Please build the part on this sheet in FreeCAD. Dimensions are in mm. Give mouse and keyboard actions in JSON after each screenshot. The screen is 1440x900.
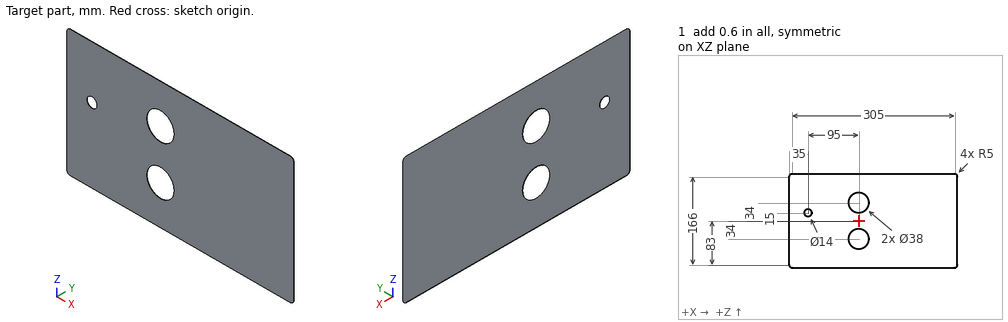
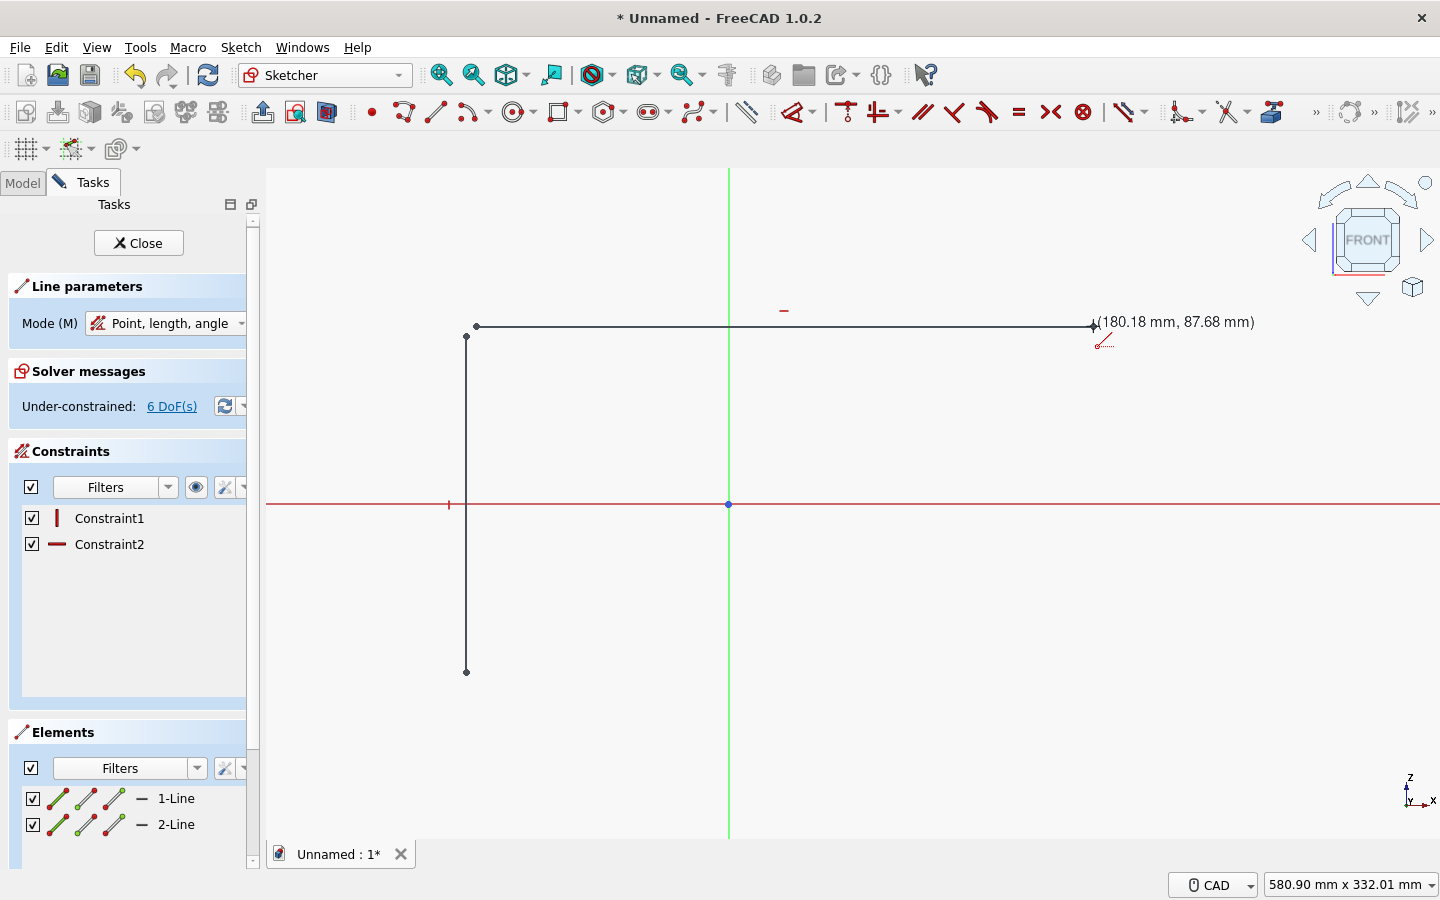
{"action": "left_click", "coordinate": [1103, 336]}
{"action": "left_click", "coordinate": [1103, 672]}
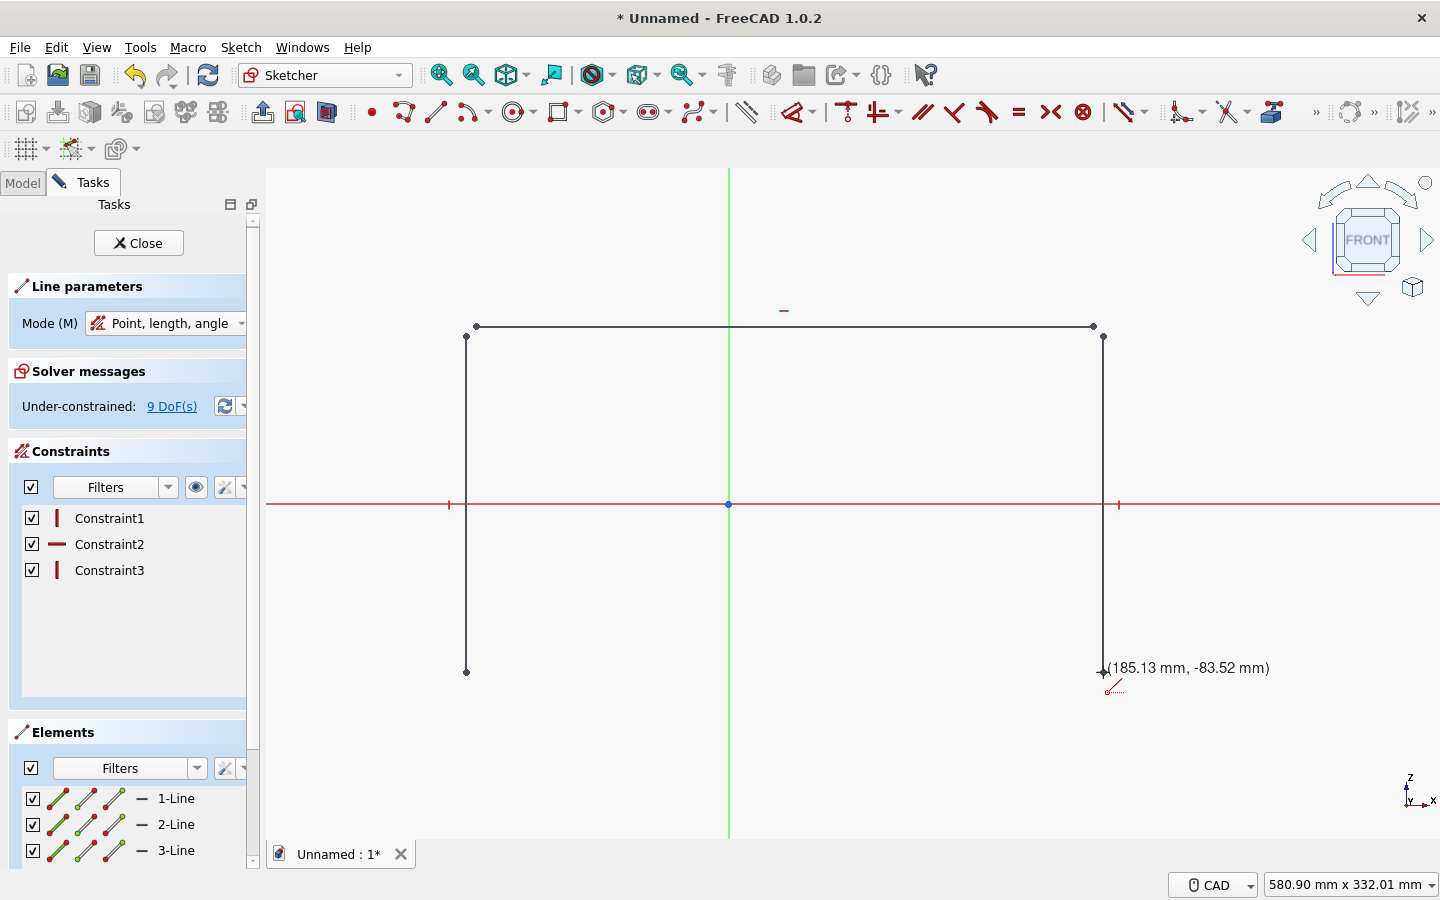
{"action": "left_click", "coordinate": [1093, 682]}
{"action": "left_click", "coordinate": [476, 682]}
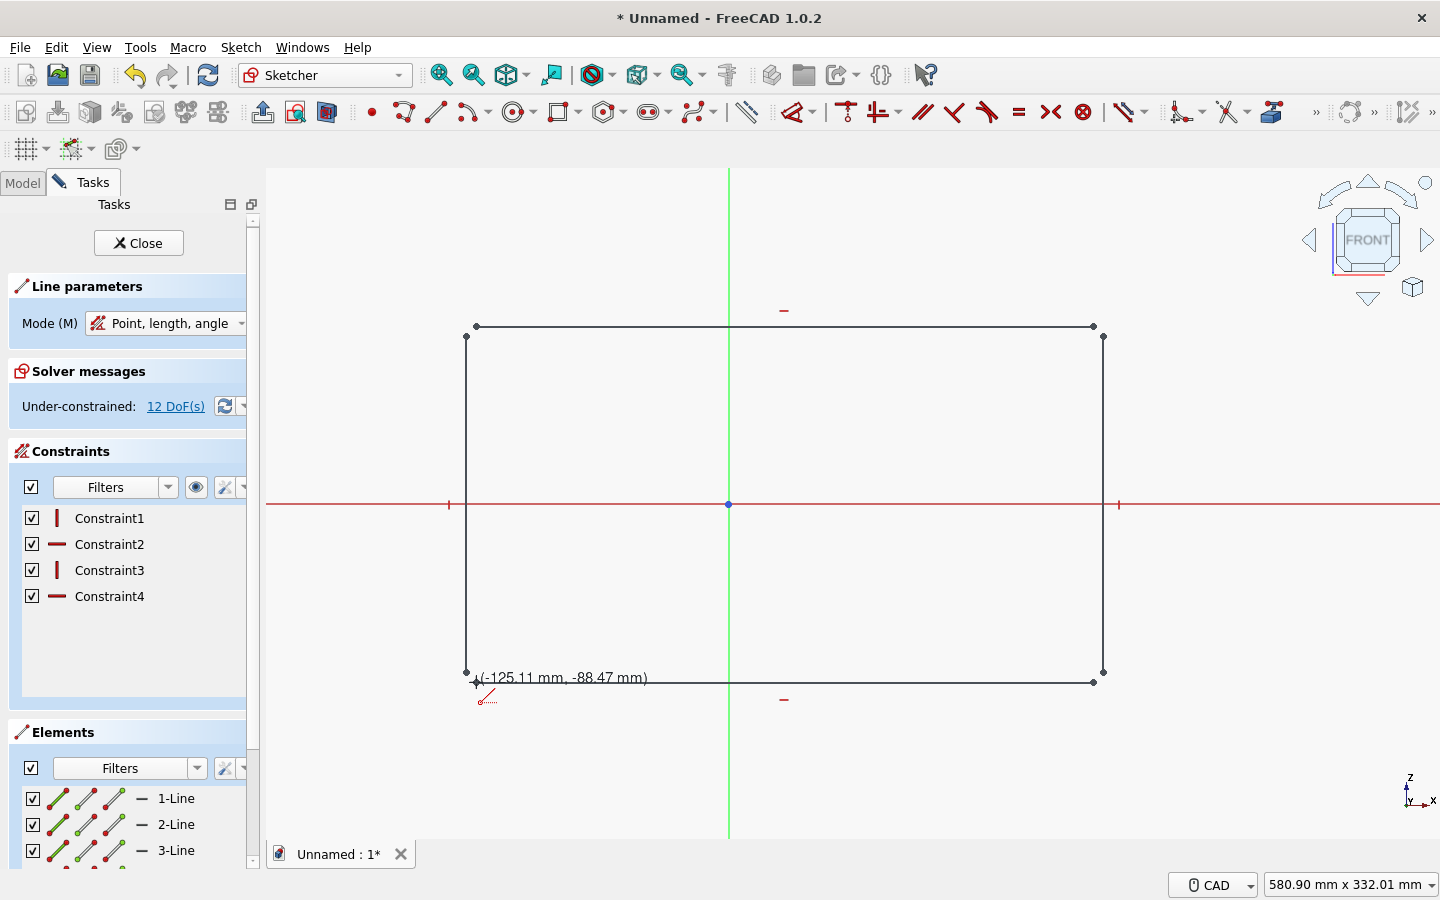
{"action": "left_click", "coordinate": [490, 112]}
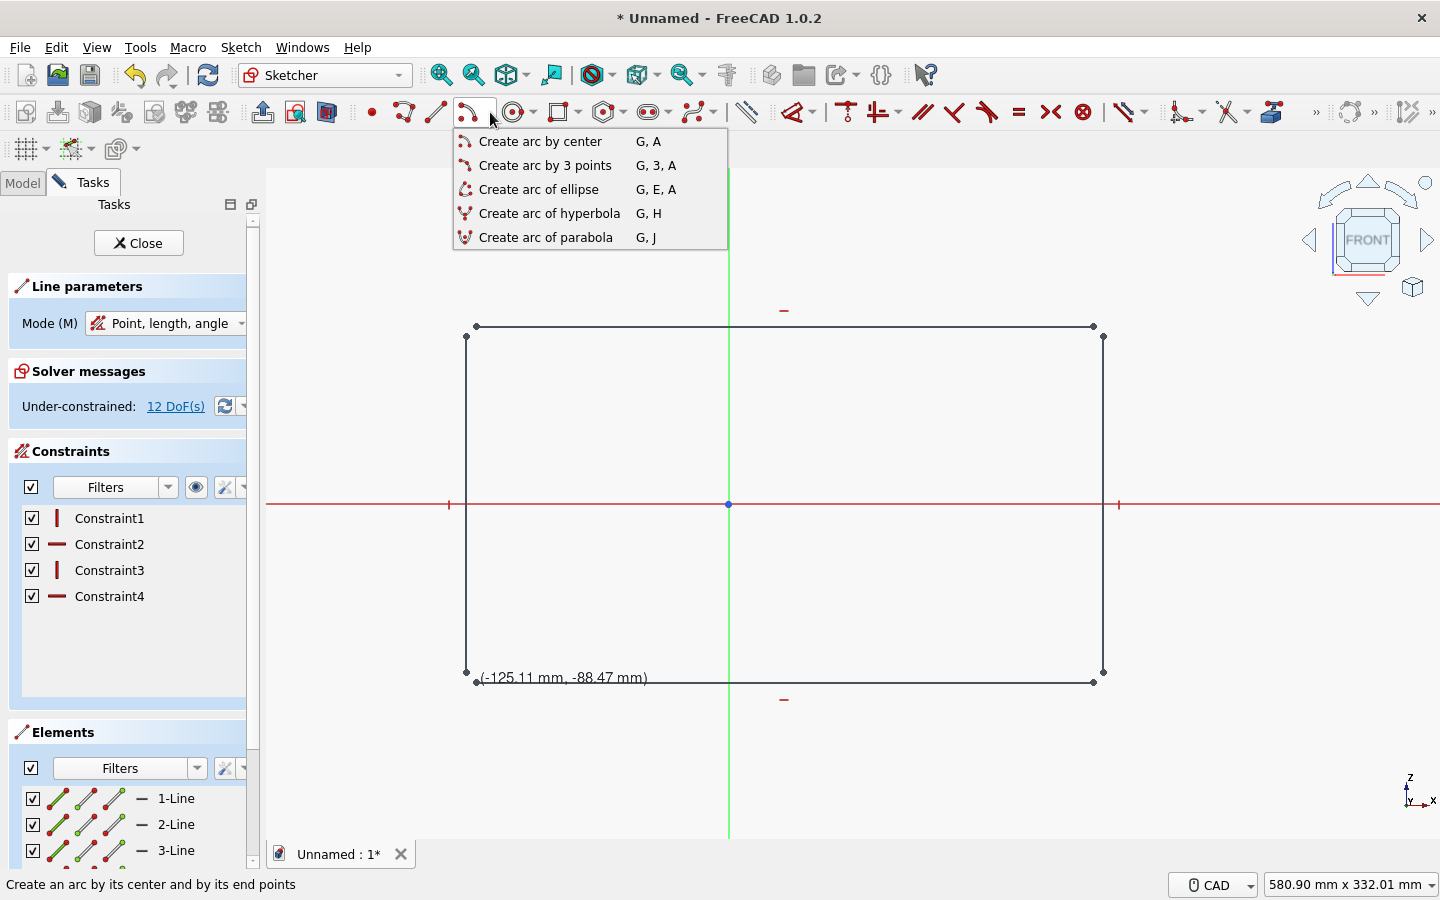
{"action": "left_click", "coordinate": [590, 165]}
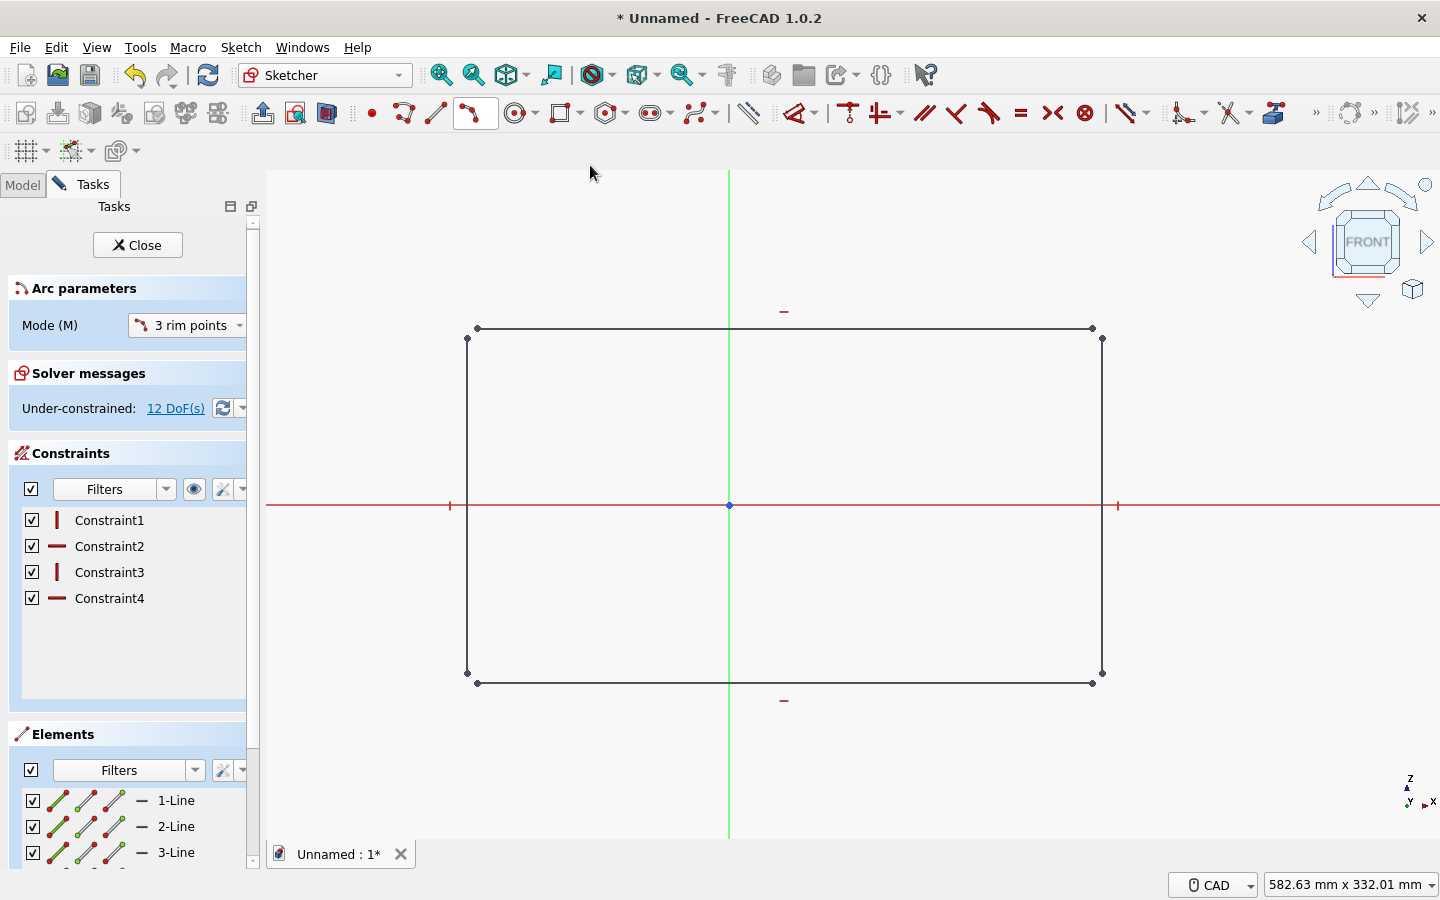
{"action": "left_click", "coordinate": [467, 338]}
{"action": "left_click", "coordinate": [477, 329]}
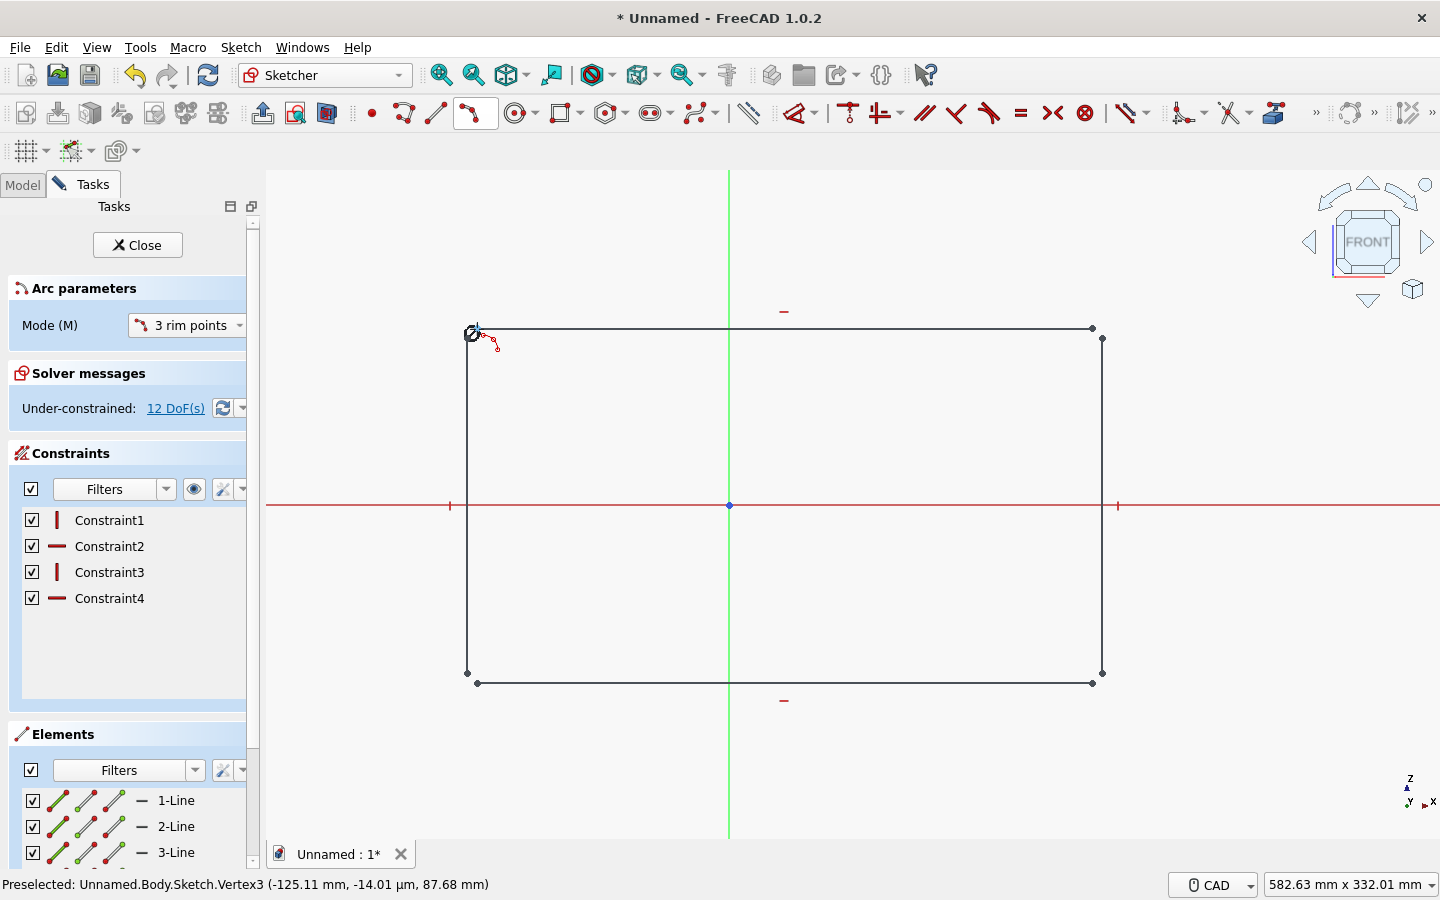
{"action": "scroll", "coordinate": [470, 331], "scroll_direction": "up", "scroll_amount": 9}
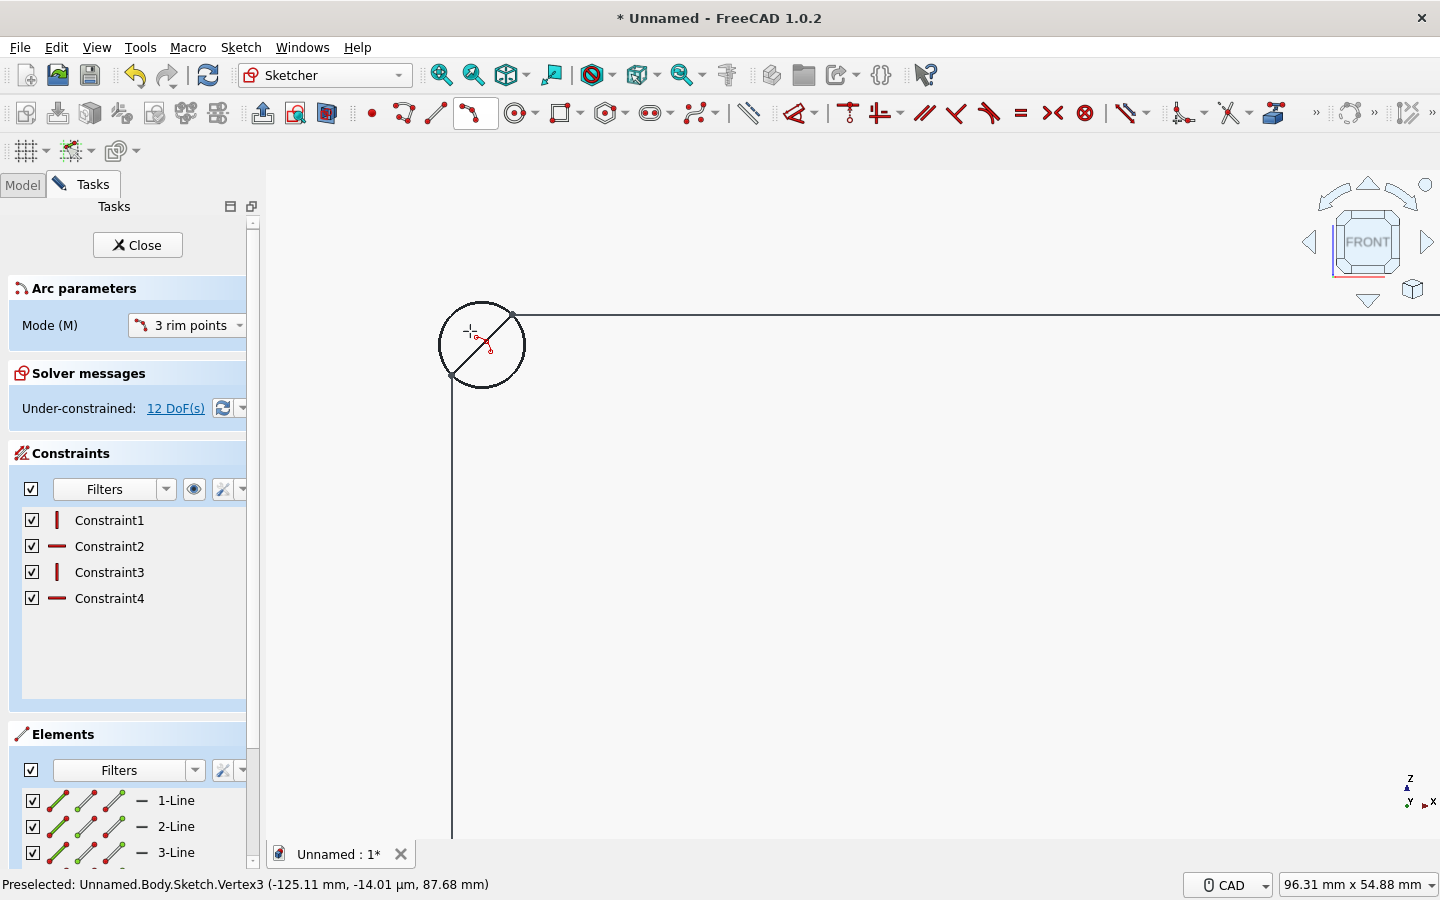
{"action": "left_click", "coordinate": [471, 329]}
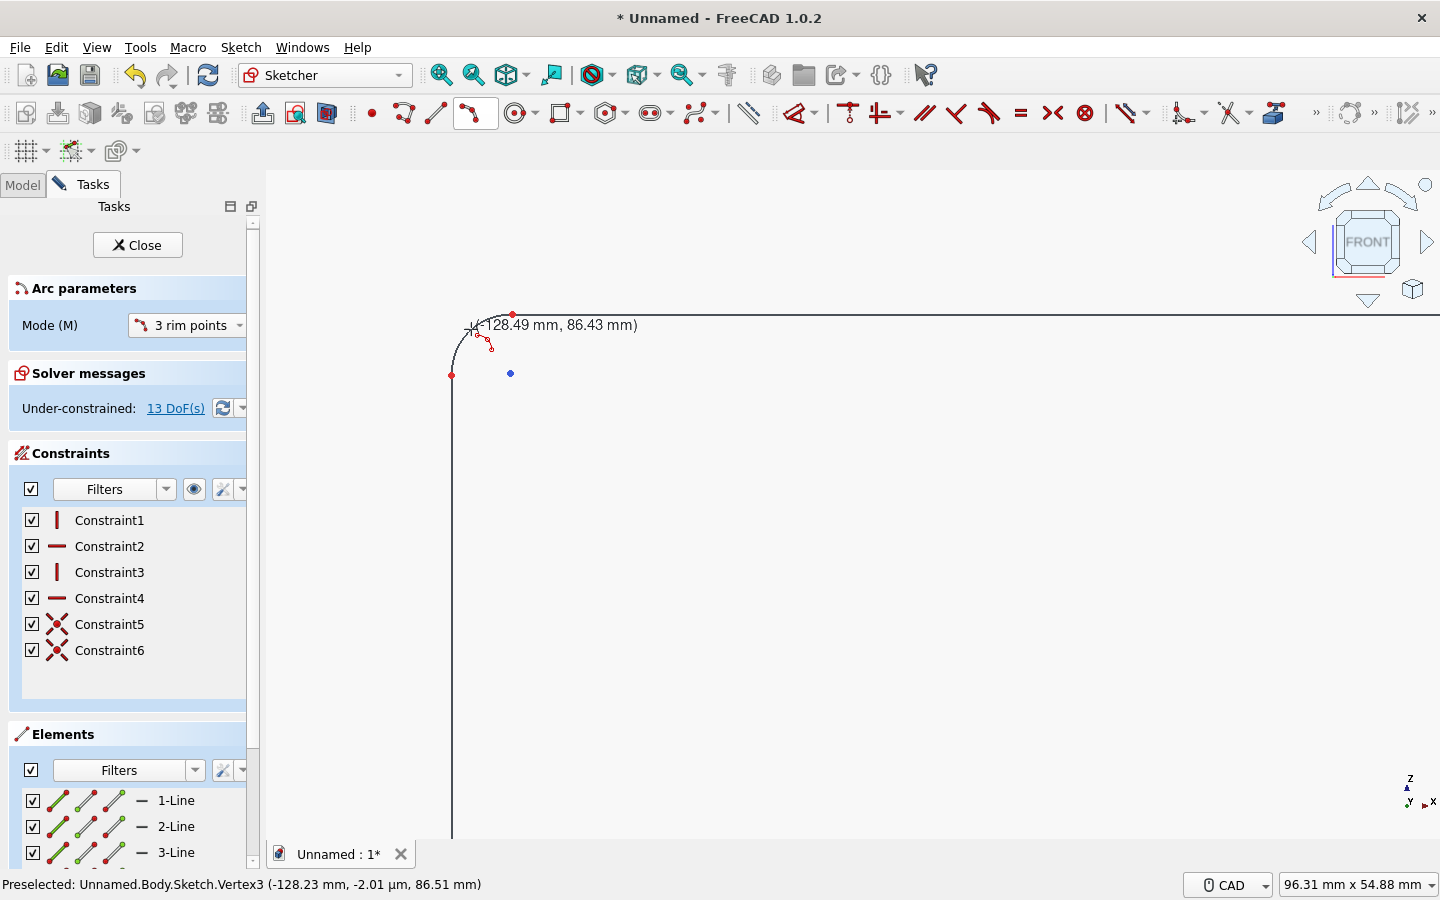
{"action": "scroll", "coordinate": [470, 330], "scroll_direction": "down", "scroll_amount": 9}